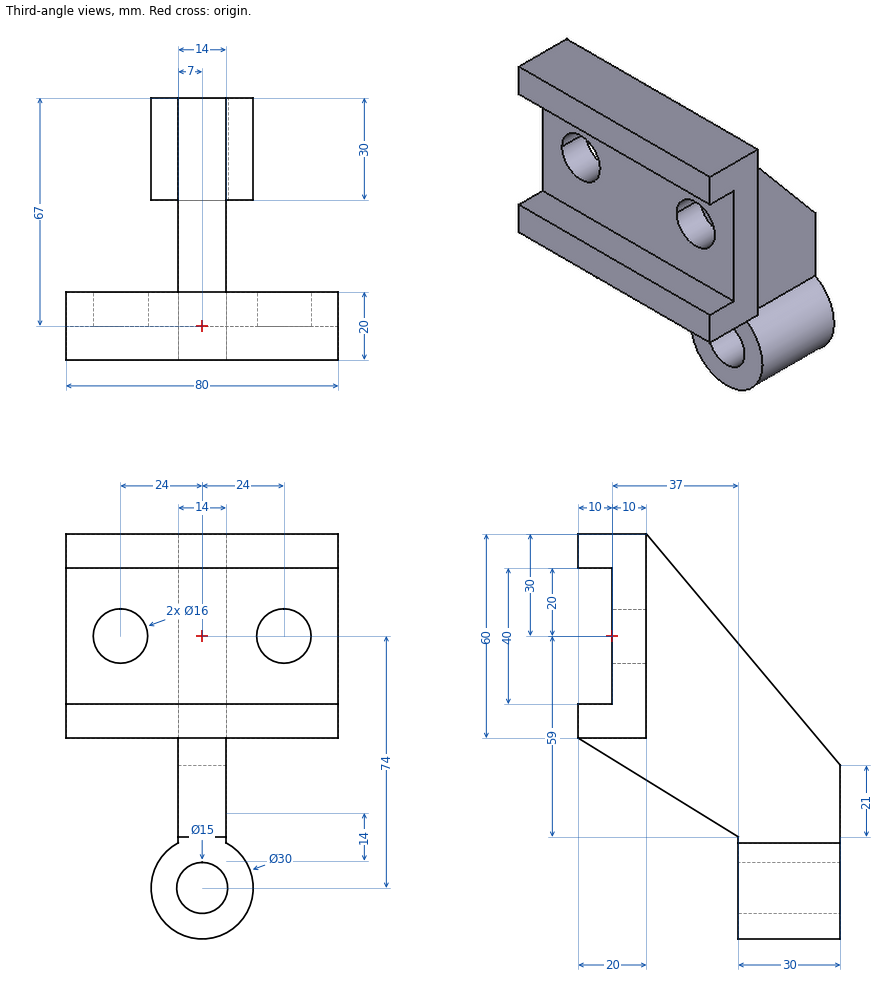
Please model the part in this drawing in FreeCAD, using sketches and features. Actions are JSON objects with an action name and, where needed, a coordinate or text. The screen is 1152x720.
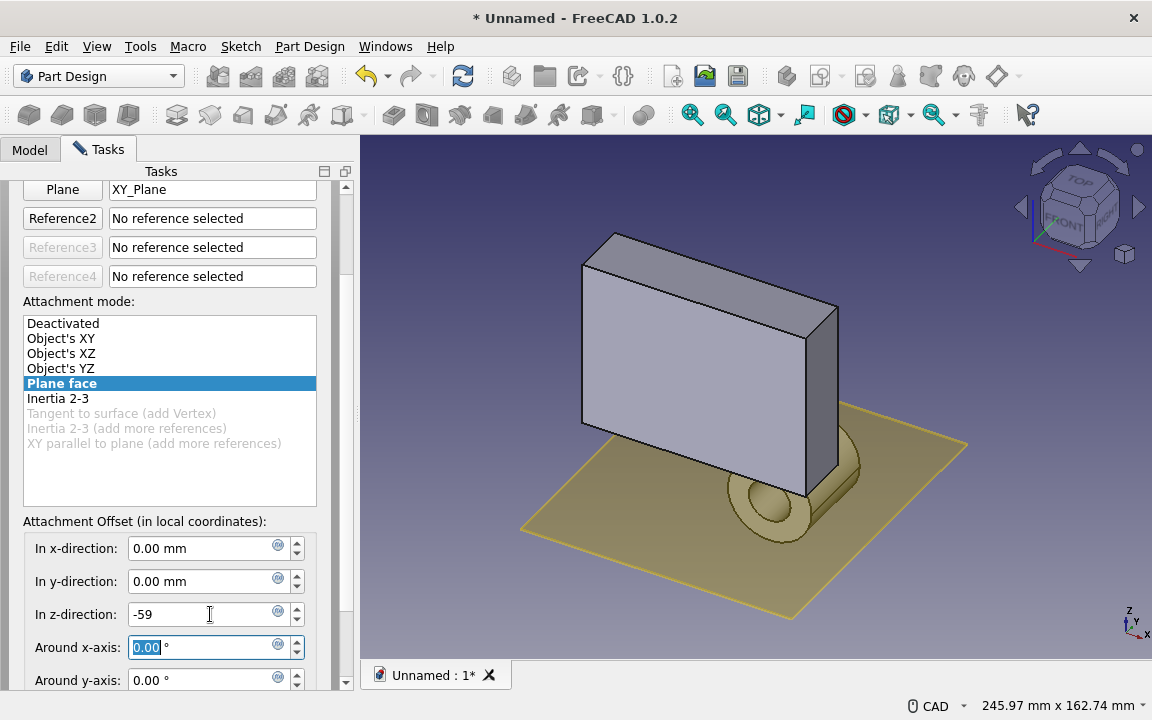
{"action": "scroll", "coordinate": [346, 436], "scroll_direction": "up", "scroll_amount": 3}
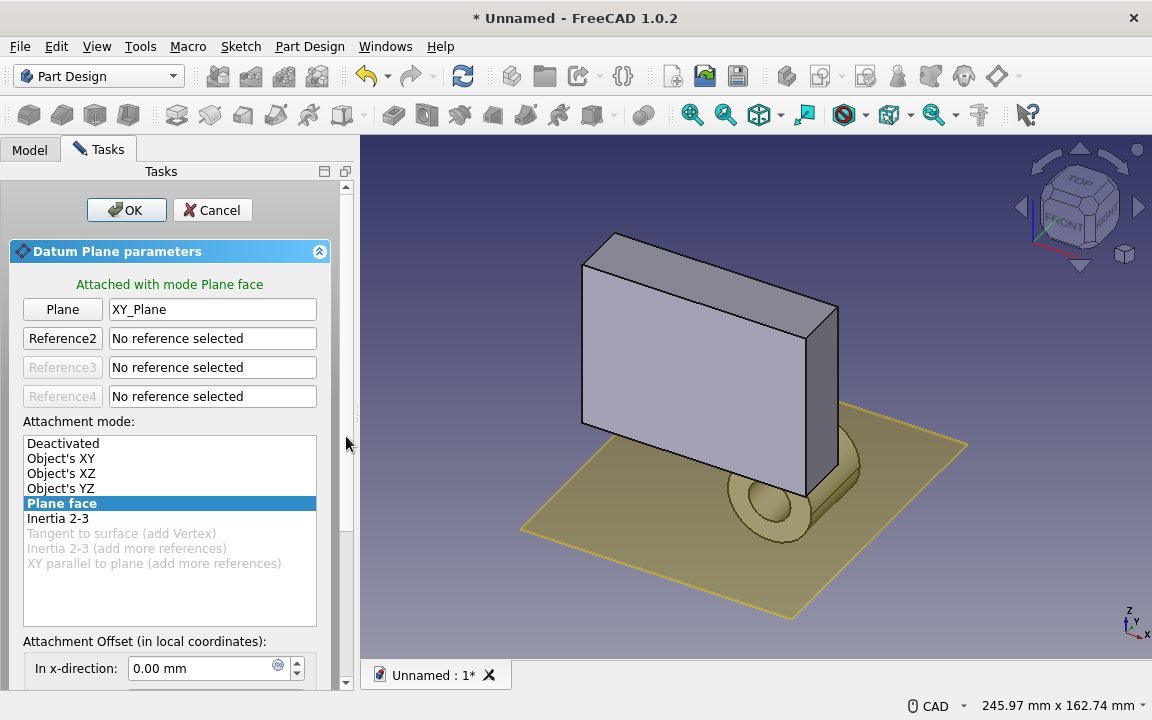
{"action": "left_click", "coordinate": [127, 210]}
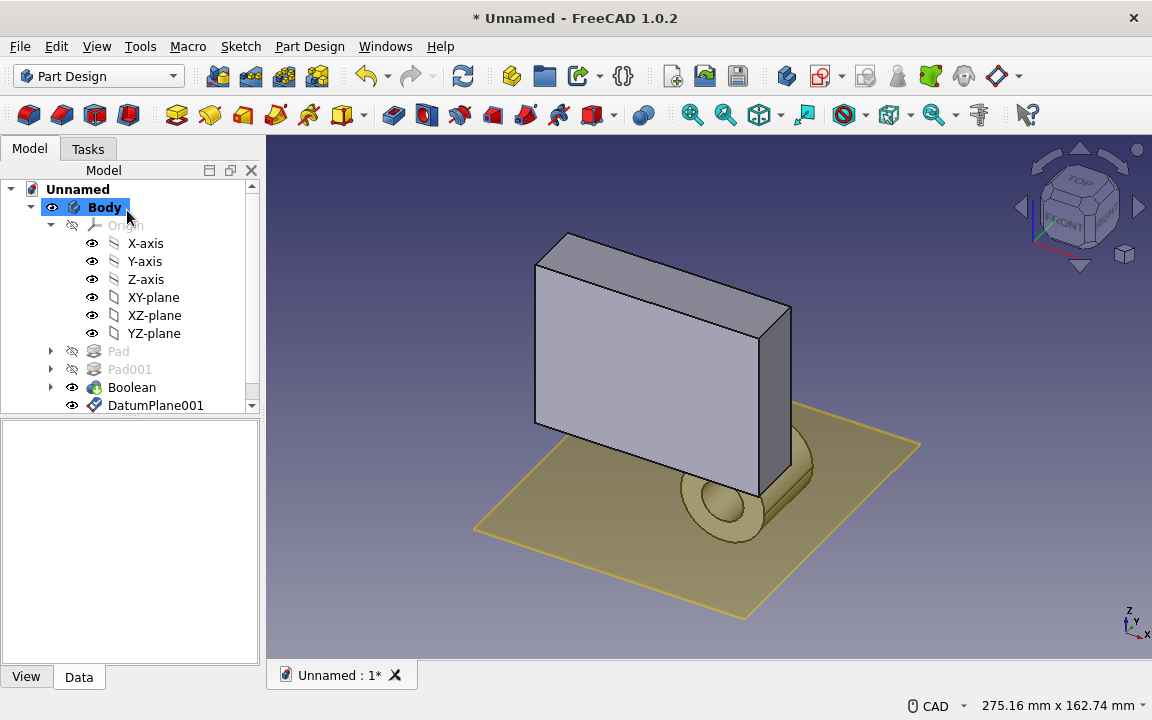
{"action": "left_click", "coordinate": [117, 405]}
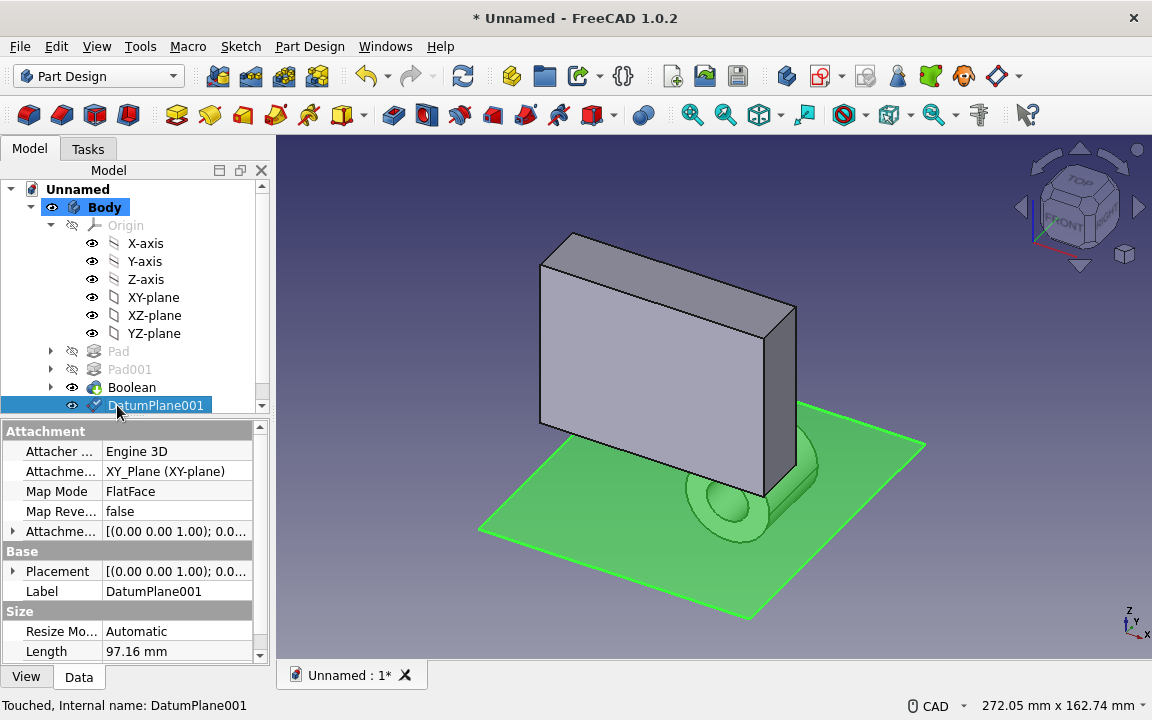
{"action": "left_click", "coordinate": [820, 76]}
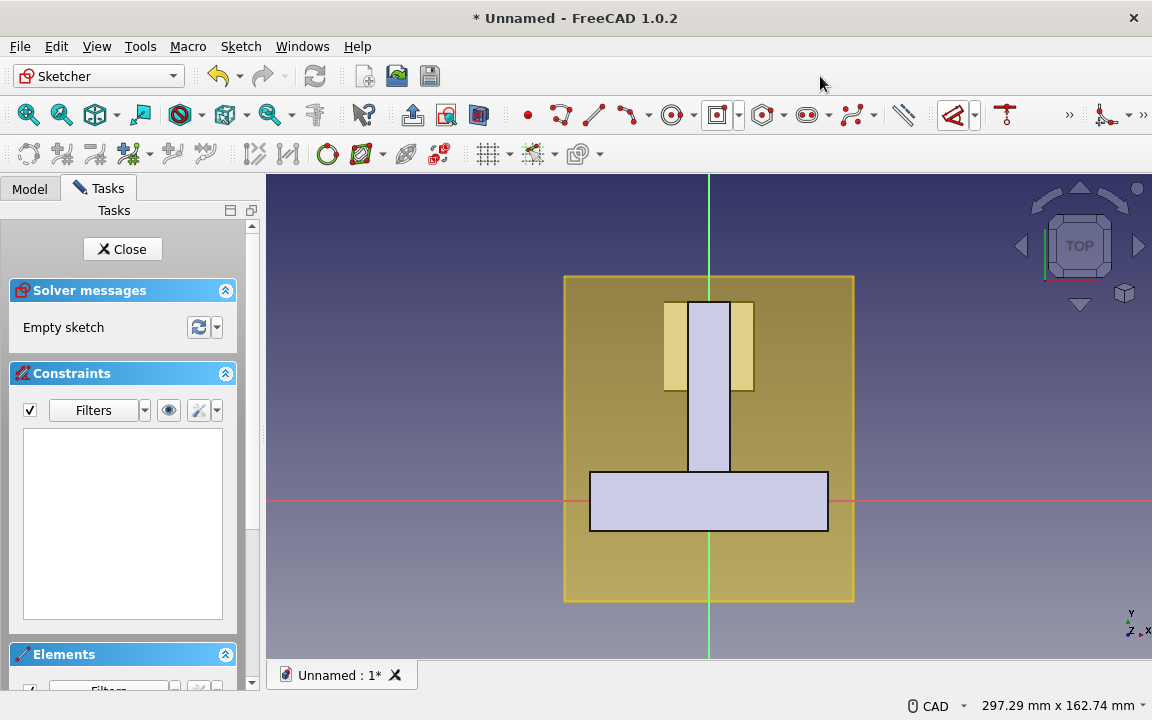
{"action": "left_click", "coordinate": [479, 116]}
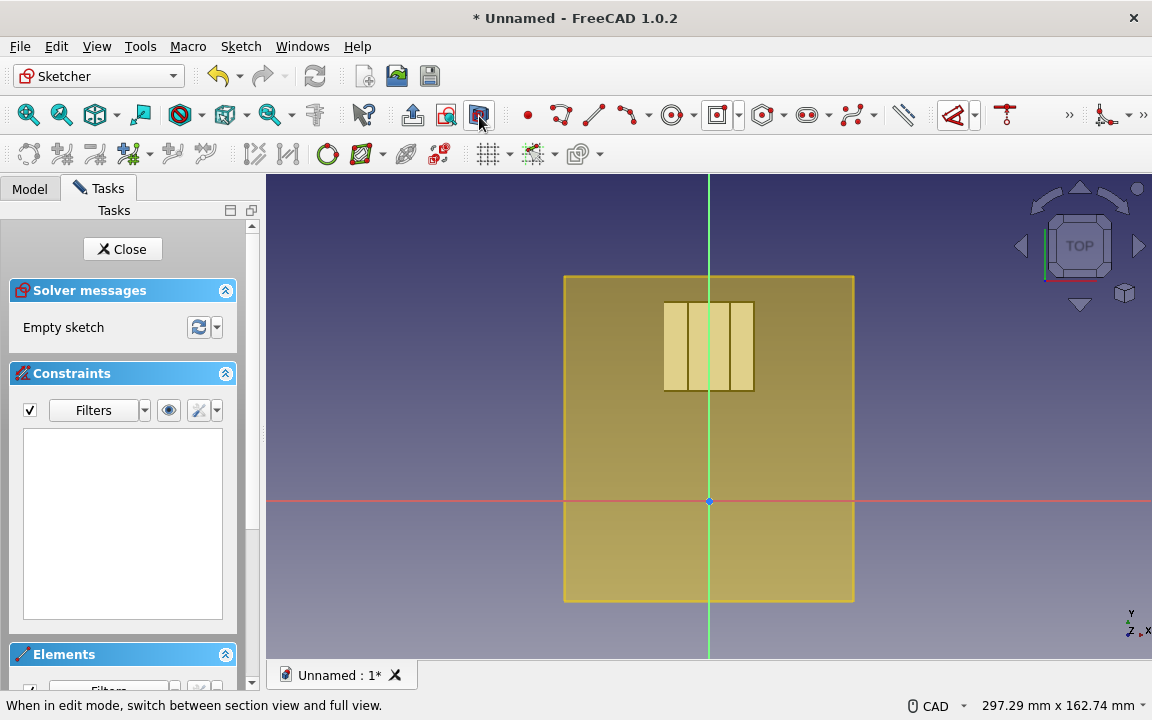
{"action": "scroll", "coordinate": [848, 371], "scroll_direction": "up", "scroll_amount": 2}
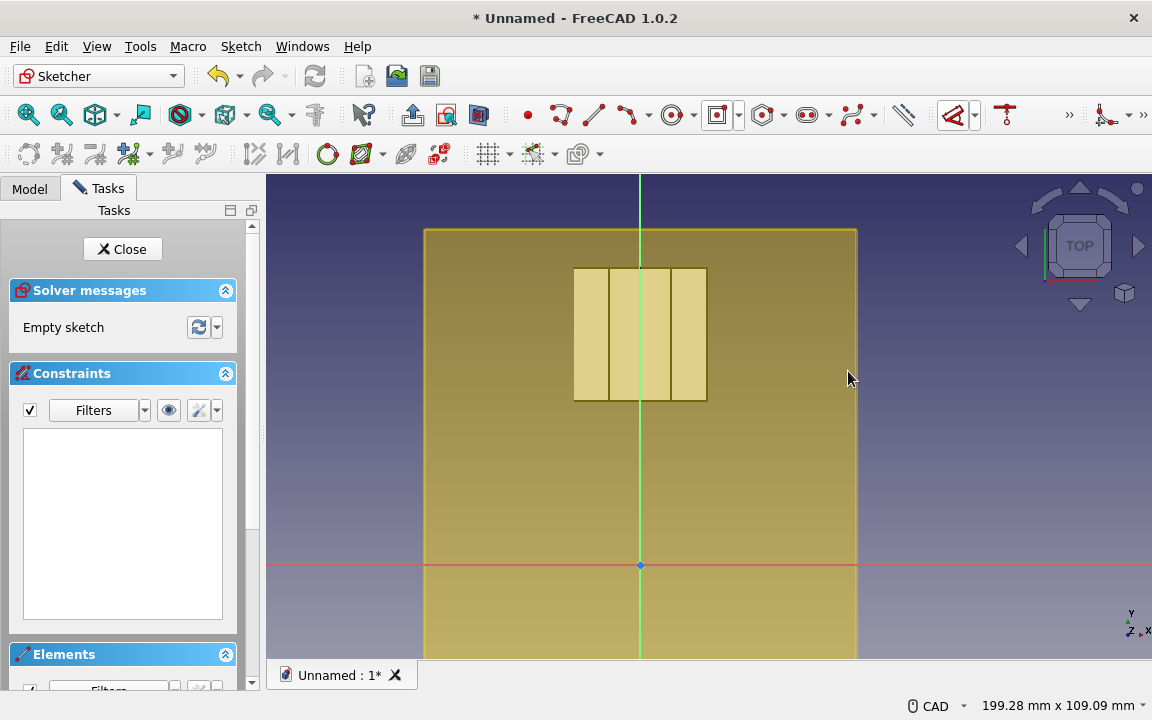
{"action": "left_click", "coordinate": [738, 116]}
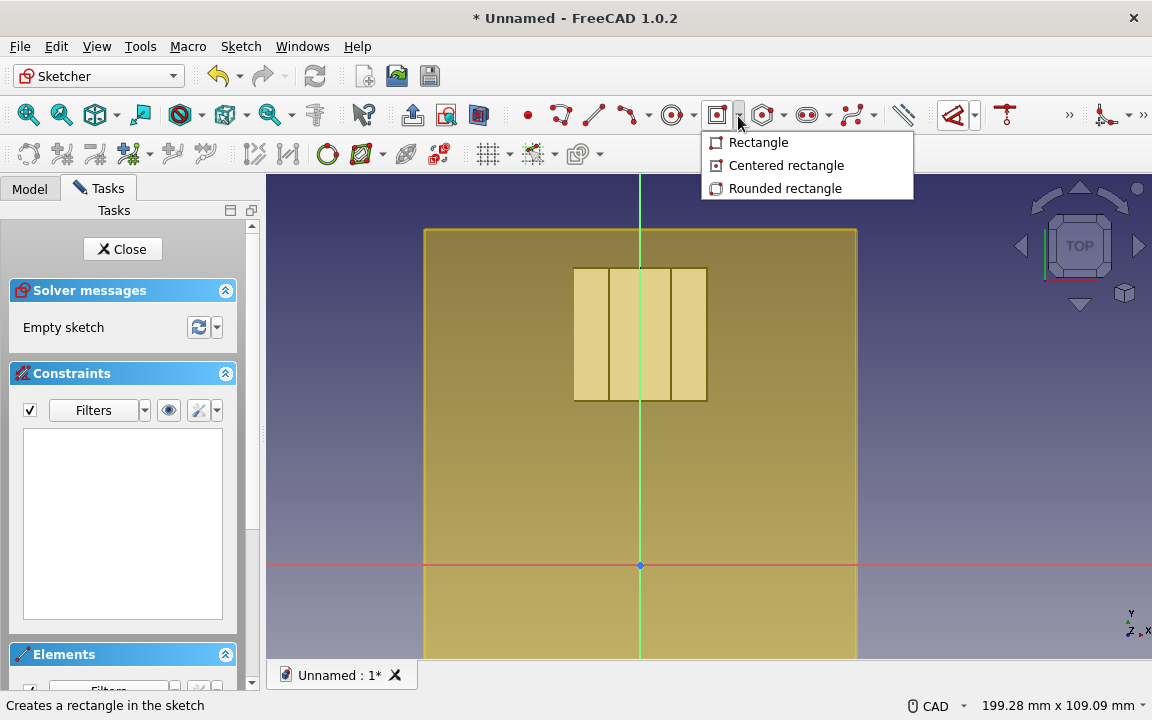
{"action": "left_click", "coordinate": [808, 142]}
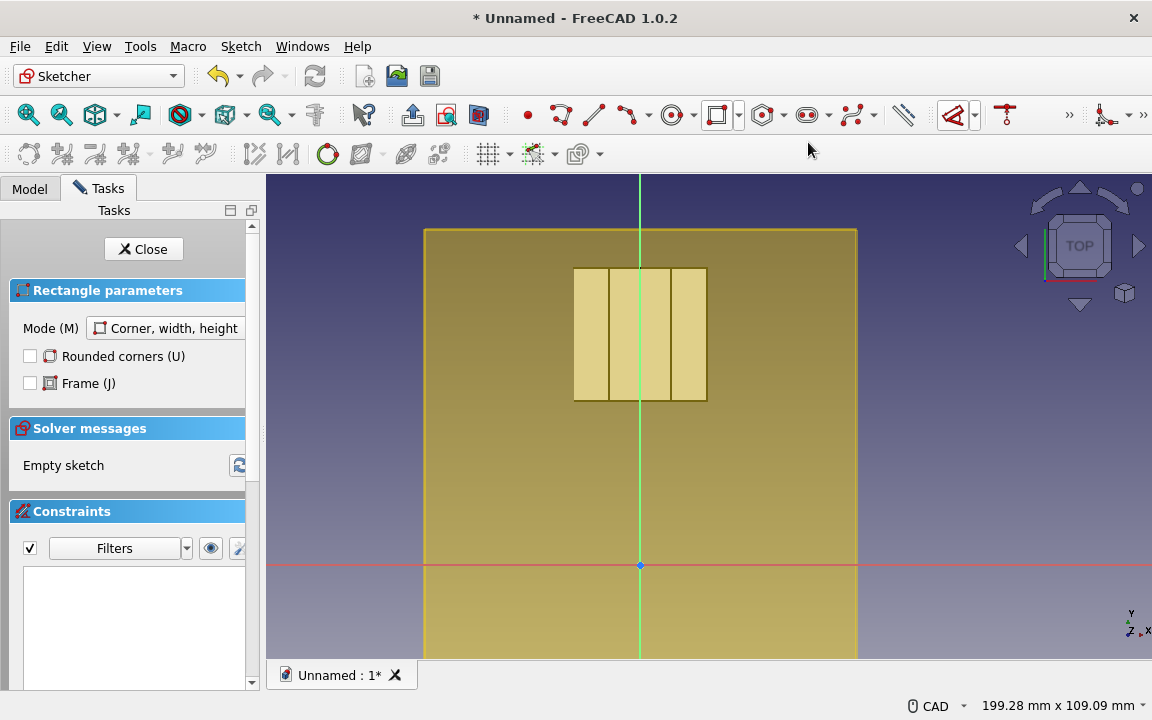
{"action": "left_click", "coordinate": [609, 268]}
{"action": "mouse_move", "coordinate": [671, 401]}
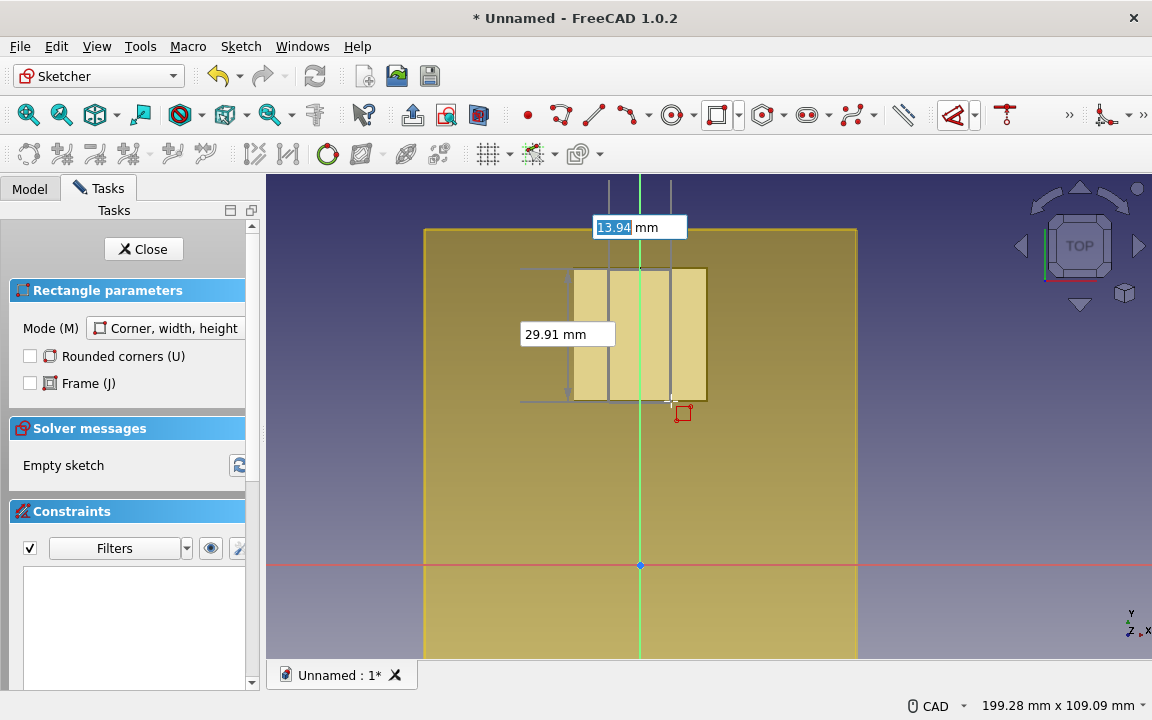
{"action": "type", "text": "14"}
{"action": "key", "text": "Tab"}
{"action": "type", "text": "30"}
{"action": "key", "text": "Return"}
{"action": "key", "text": "Escape"}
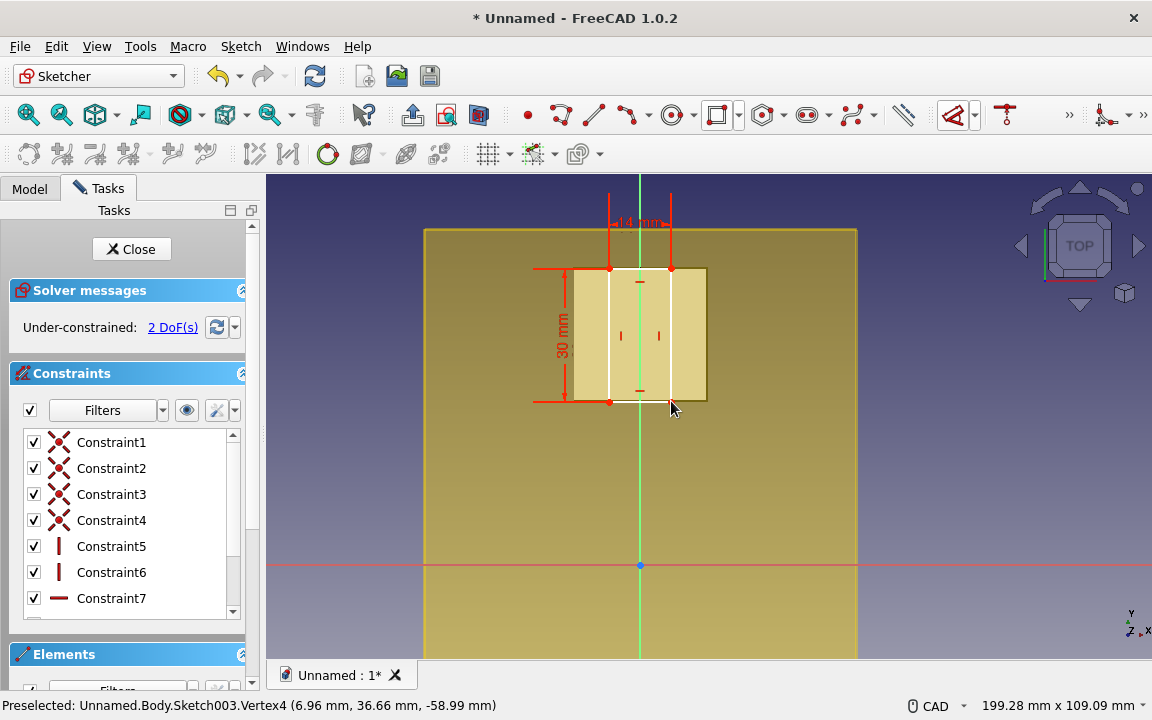
{"action": "scroll", "coordinate": [609, 269], "scroll_direction": "up", "scroll_amount": 2}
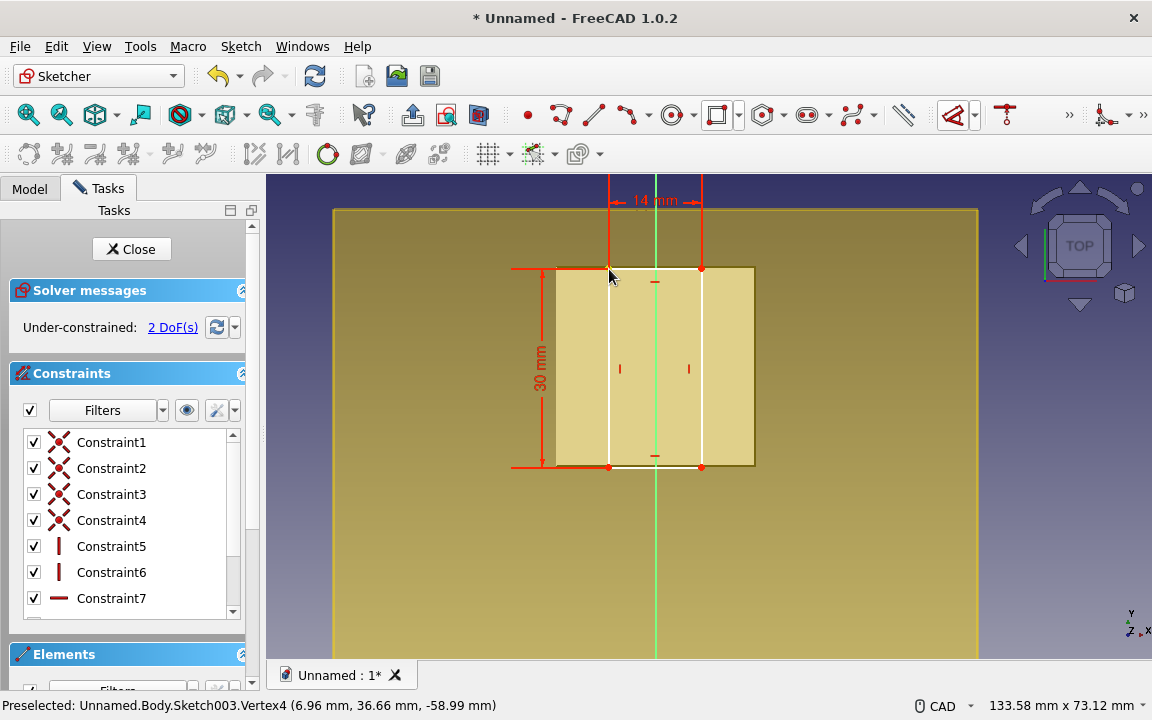
{"action": "left_click", "coordinate": [609, 269]}